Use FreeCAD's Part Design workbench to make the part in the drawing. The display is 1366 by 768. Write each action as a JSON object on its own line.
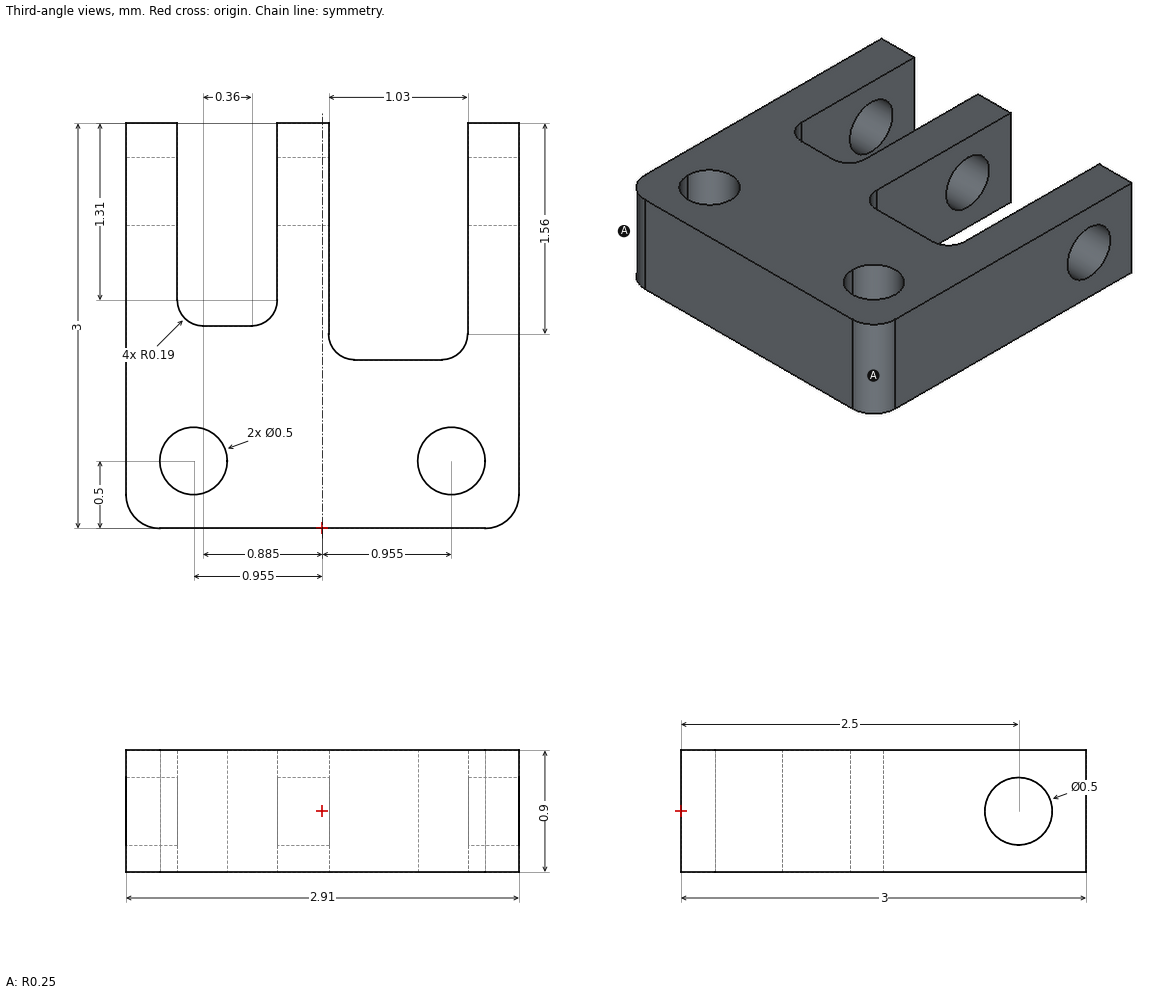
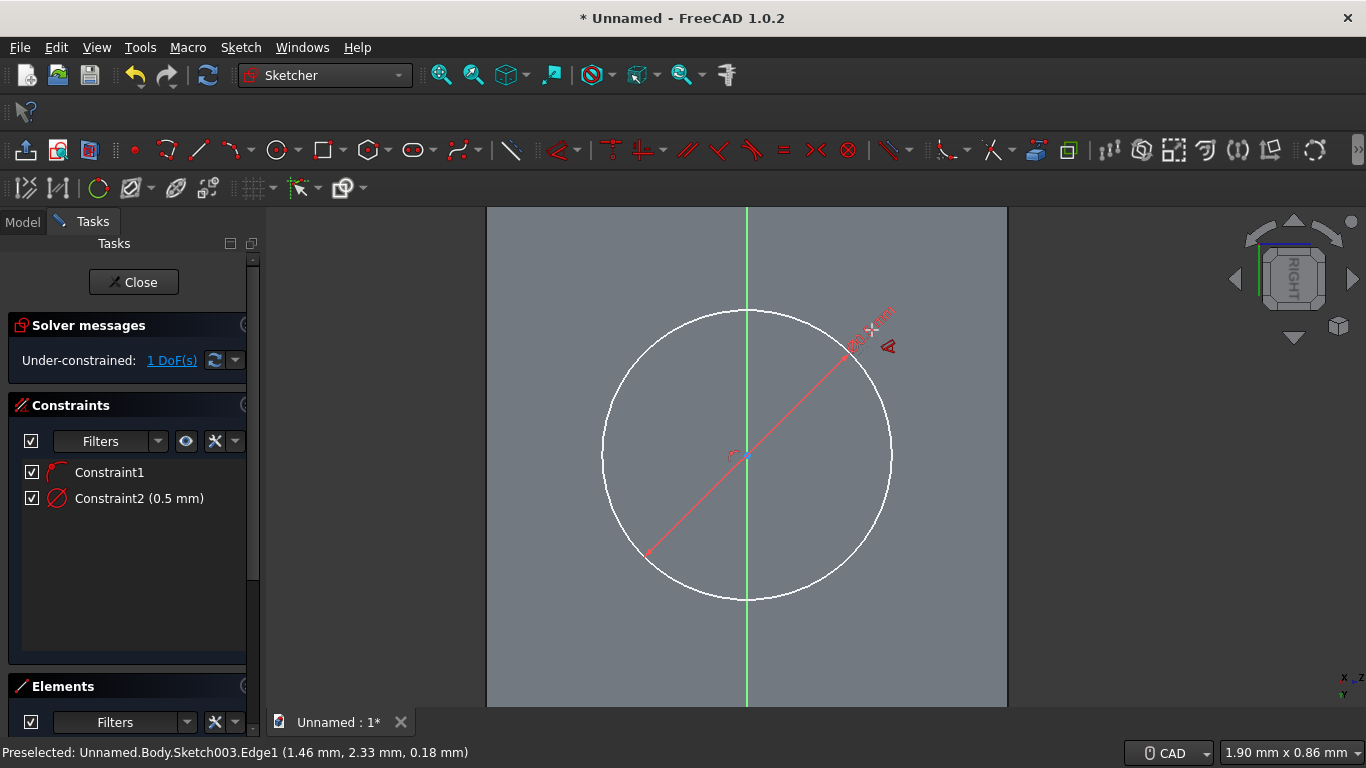
{"action": "scroll", "coordinate": [747, 455], "scroll_direction": "up", "scroll_amount": 4}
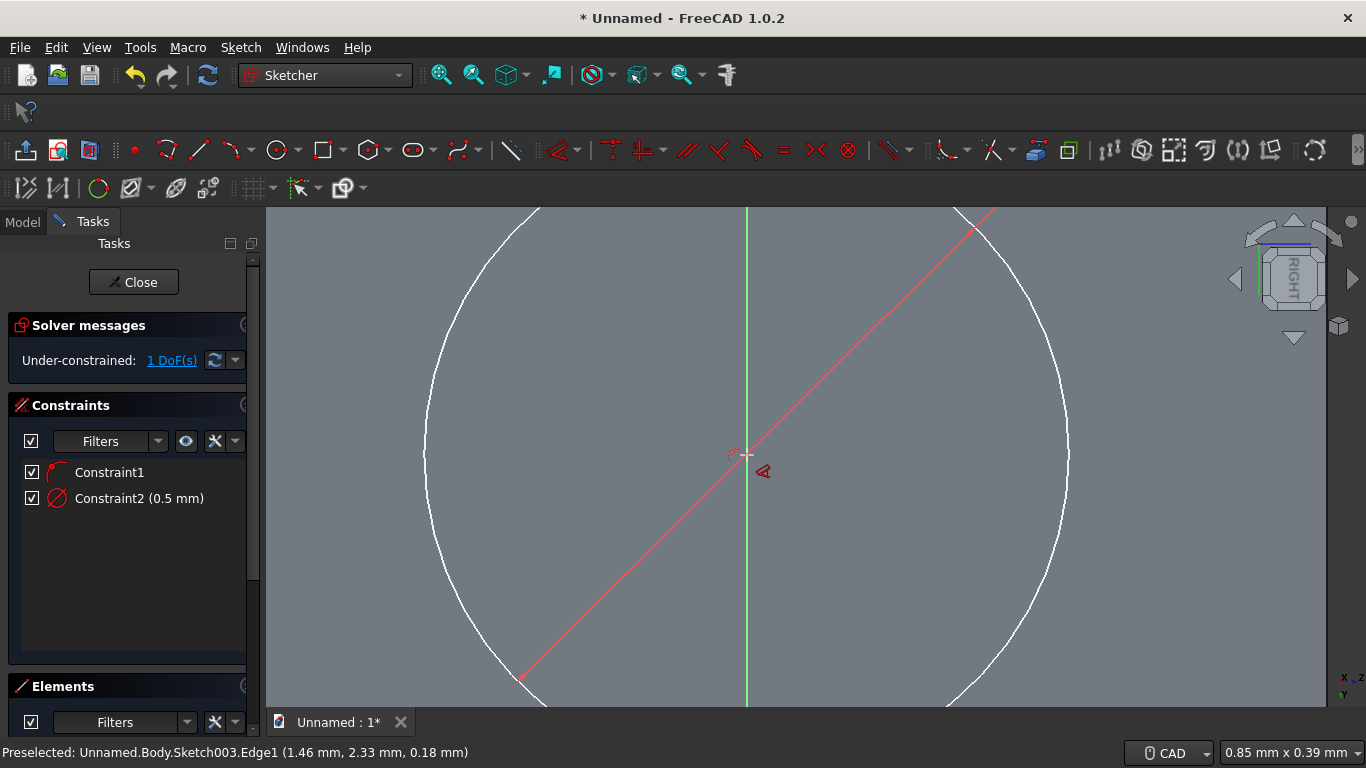
{"action": "left_click", "coordinate": [747, 454]}
{"action": "left_click", "coordinate": [781, 345]}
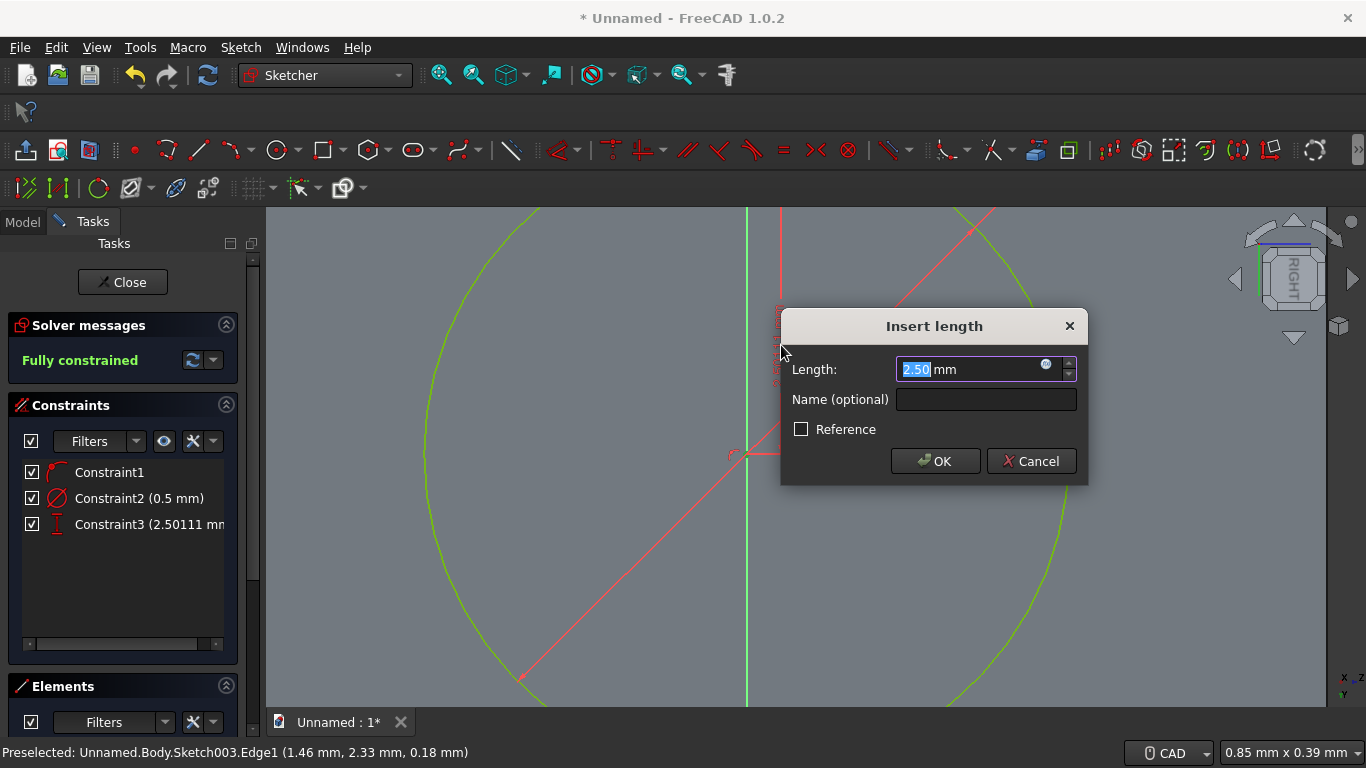
{"action": "type", "text": "2.5"}
{"action": "key", "text": "Return"}
{"action": "key", "text": "Escape"}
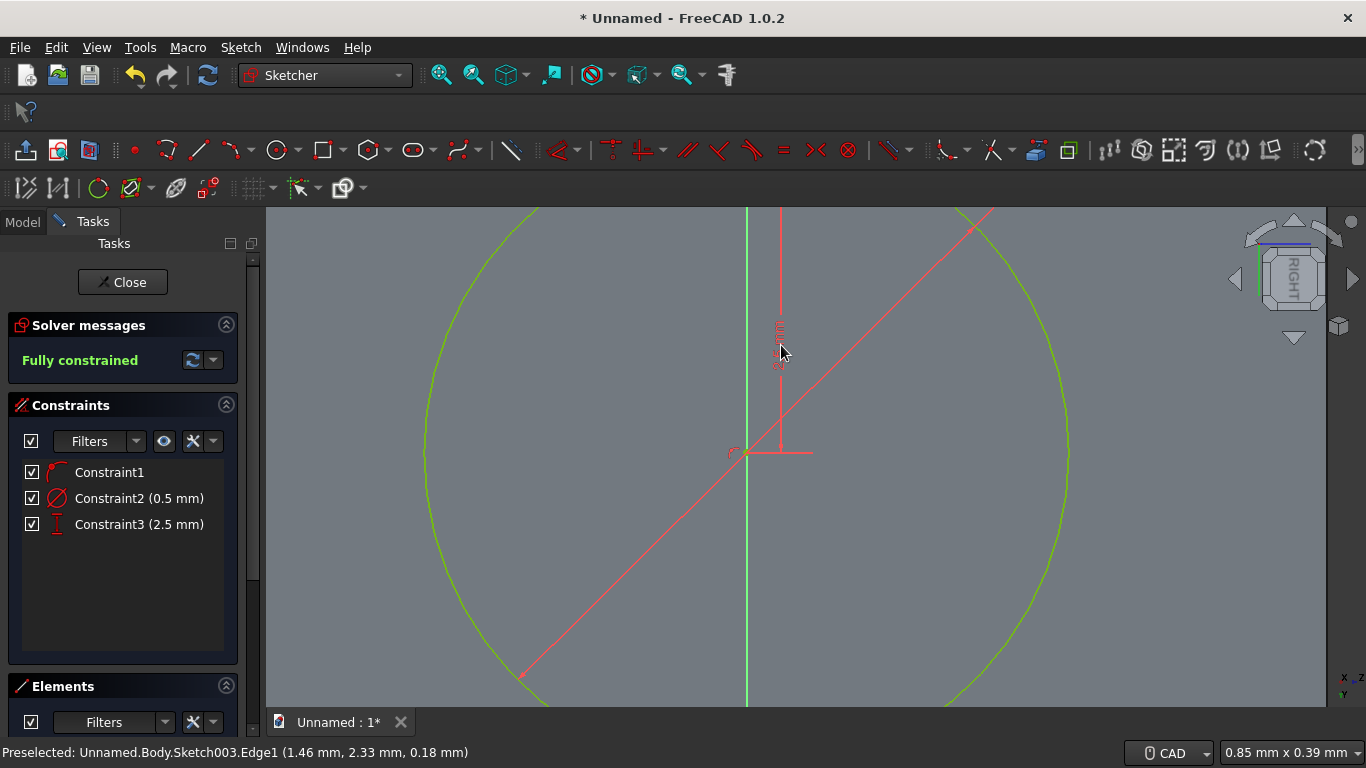
{"action": "left_click", "coordinate": [123, 282]}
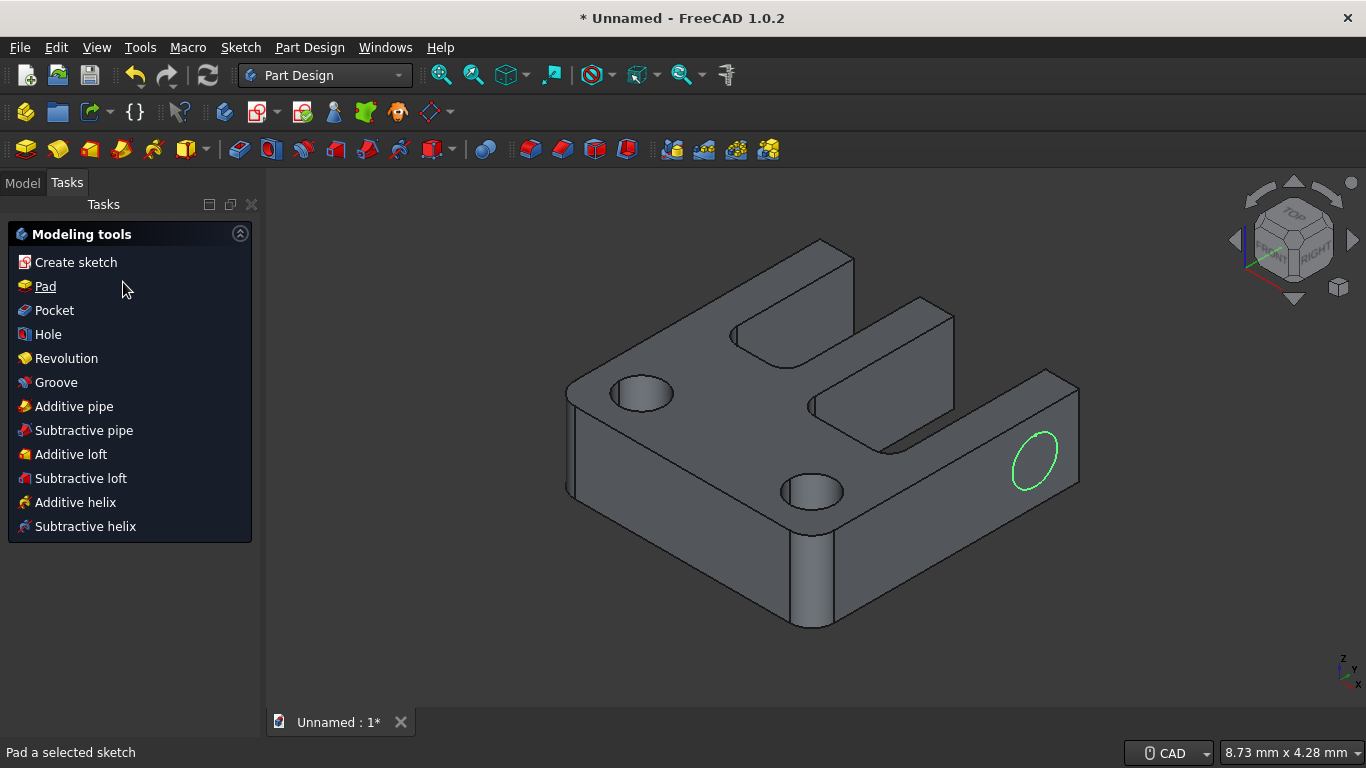
{"action": "left_click", "coordinate": [240, 150]}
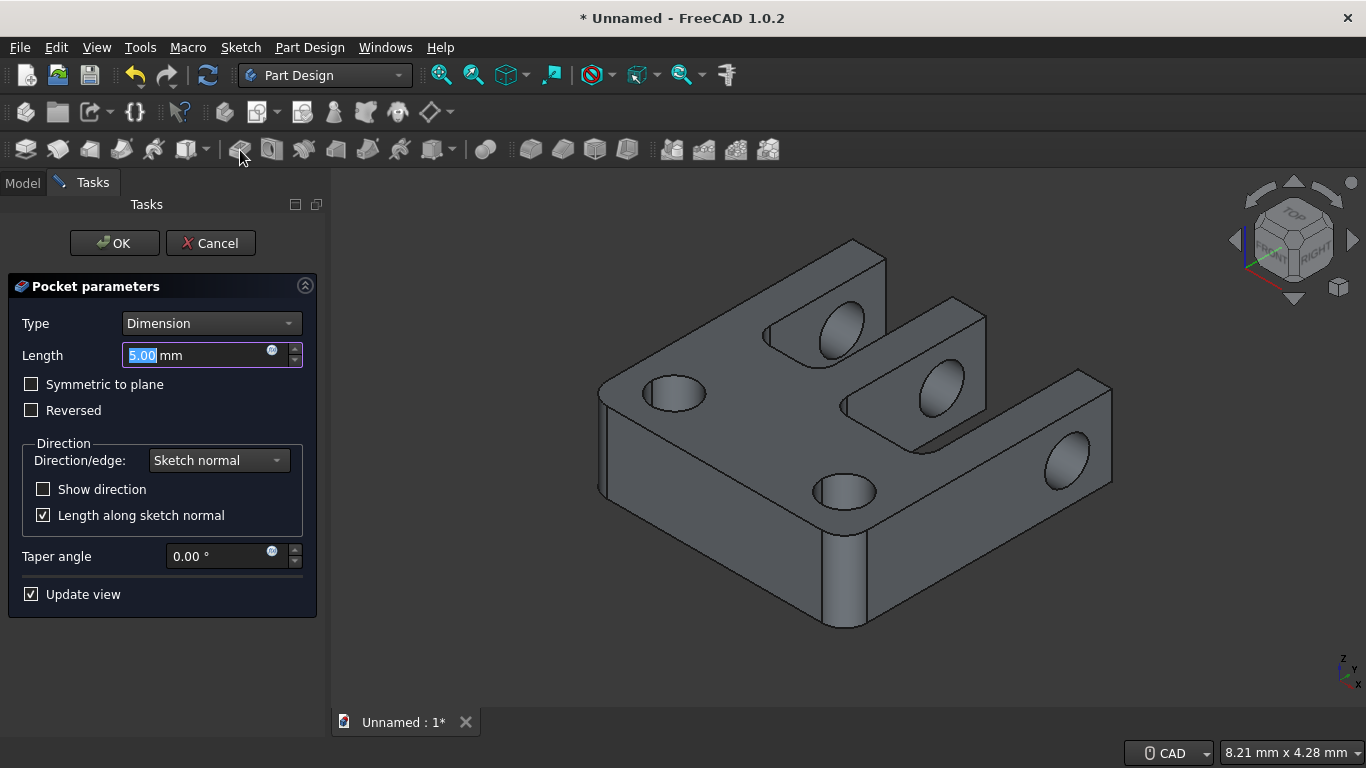
{"action": "left_click", "coordinate": [212, 324]}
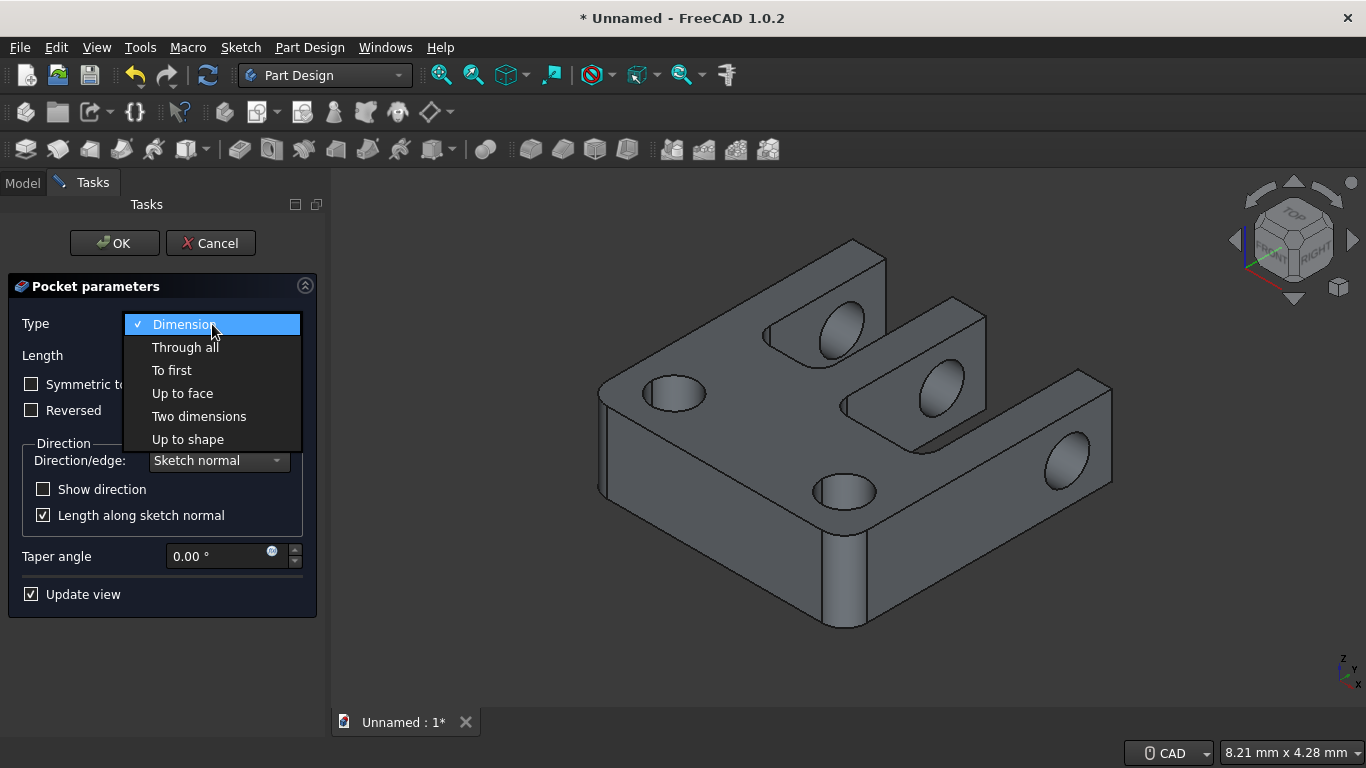
{"action": "left_click", "coordinate": [212, 348]}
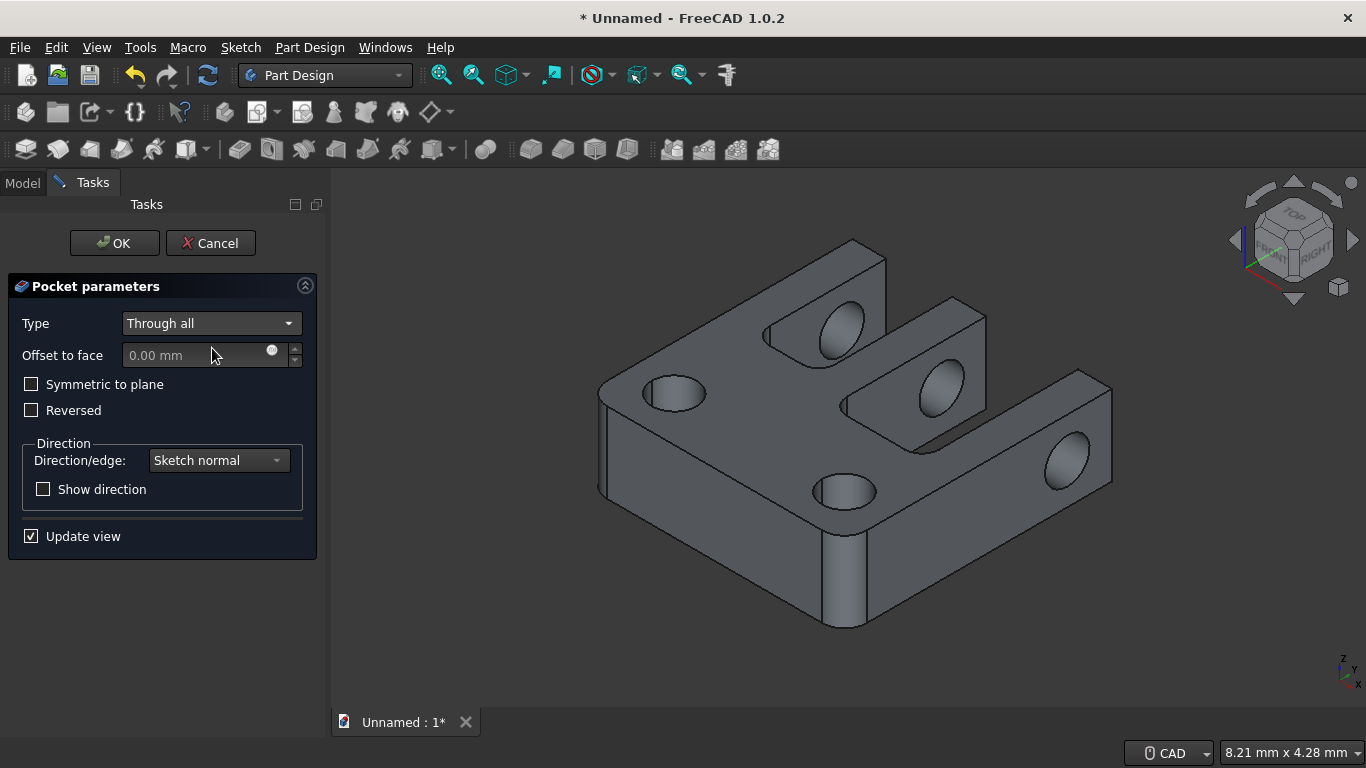
{"action": "left_click", "coordinate": [115, 243]}